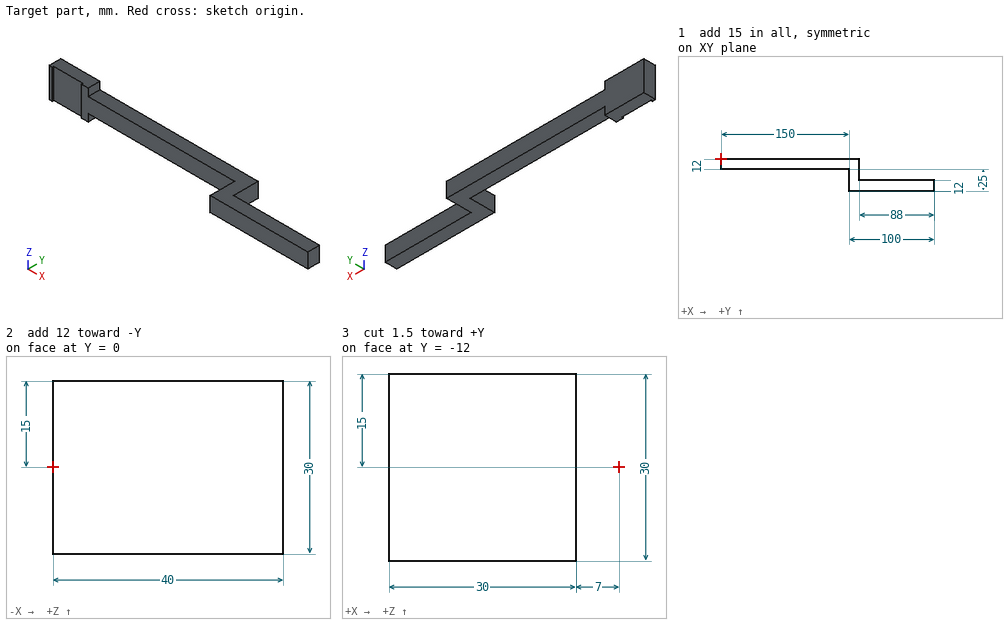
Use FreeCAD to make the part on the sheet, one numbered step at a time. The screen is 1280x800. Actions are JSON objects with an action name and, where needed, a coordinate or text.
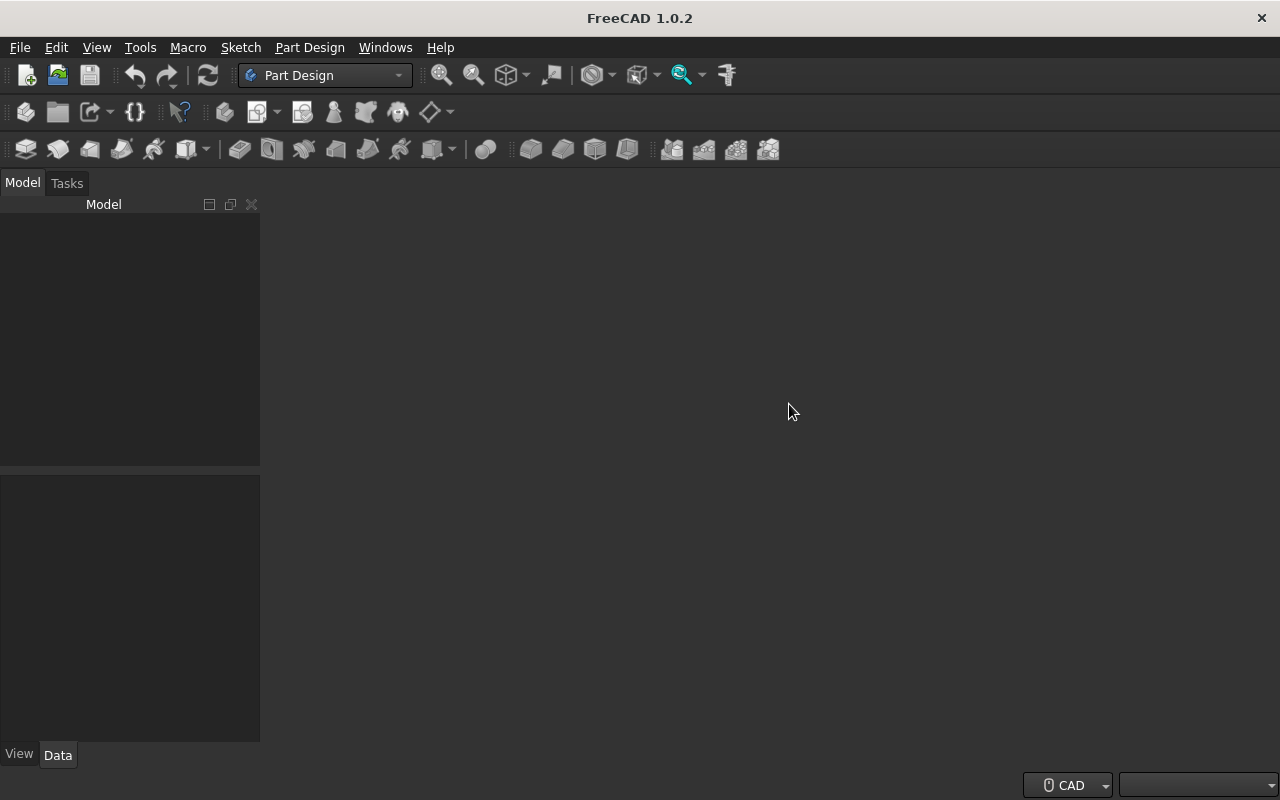
{"action": "left_click", "coordinate": [26, 76]}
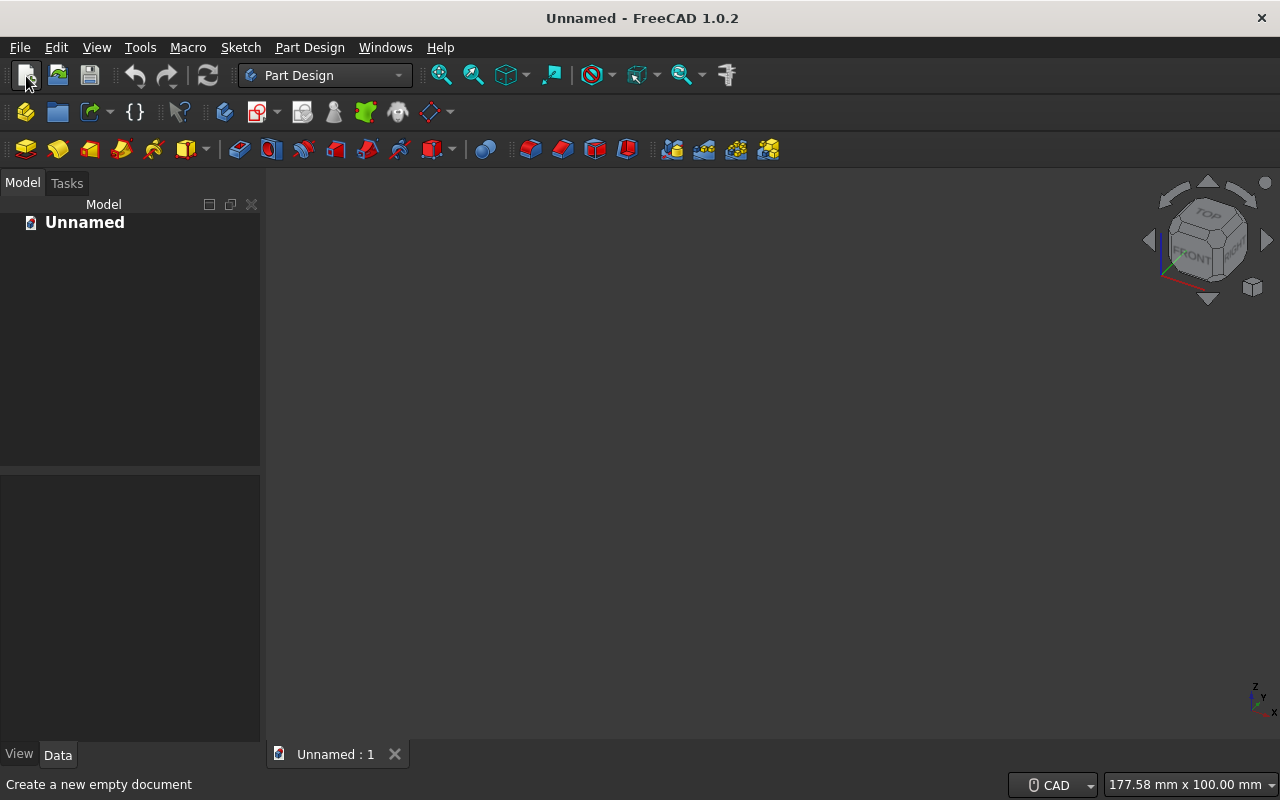
{"action": "left_click", "coordinate": [258, 112]}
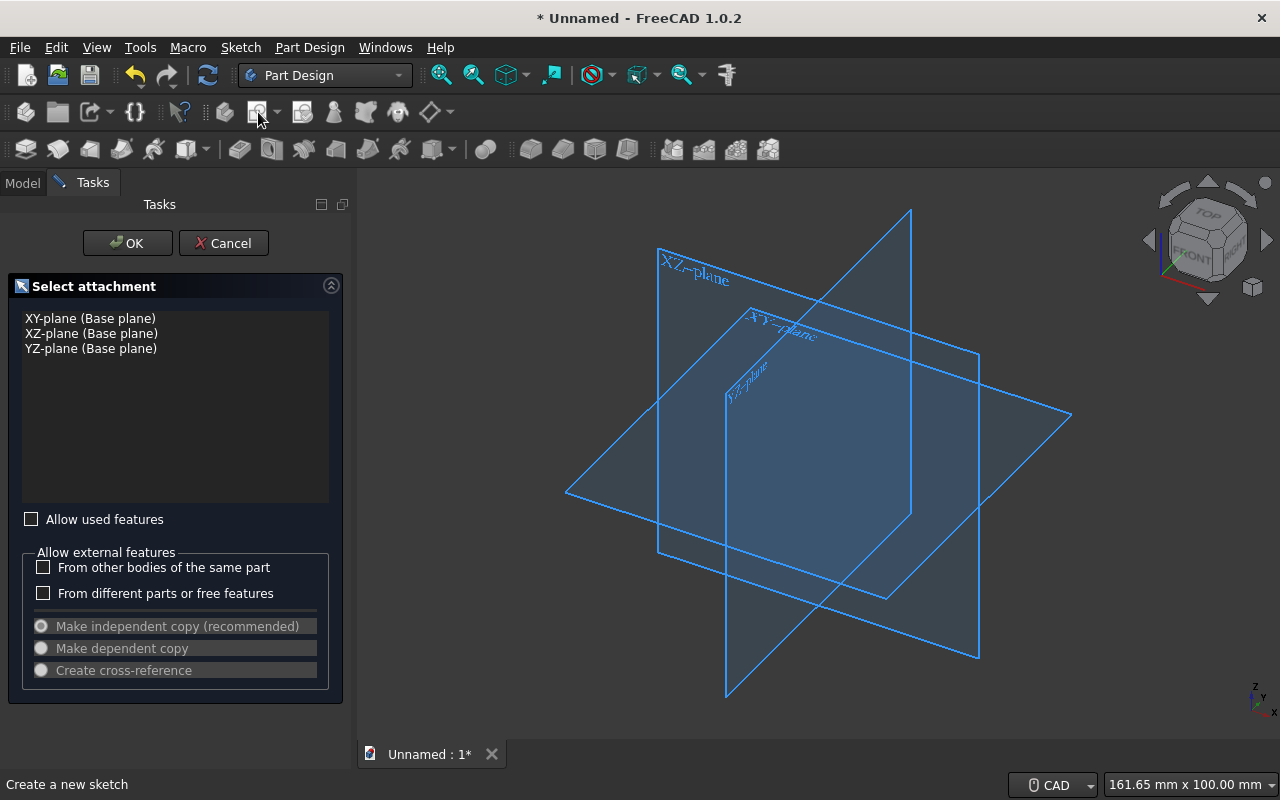
{"action": "left_click", "coordinate": [82, 318]}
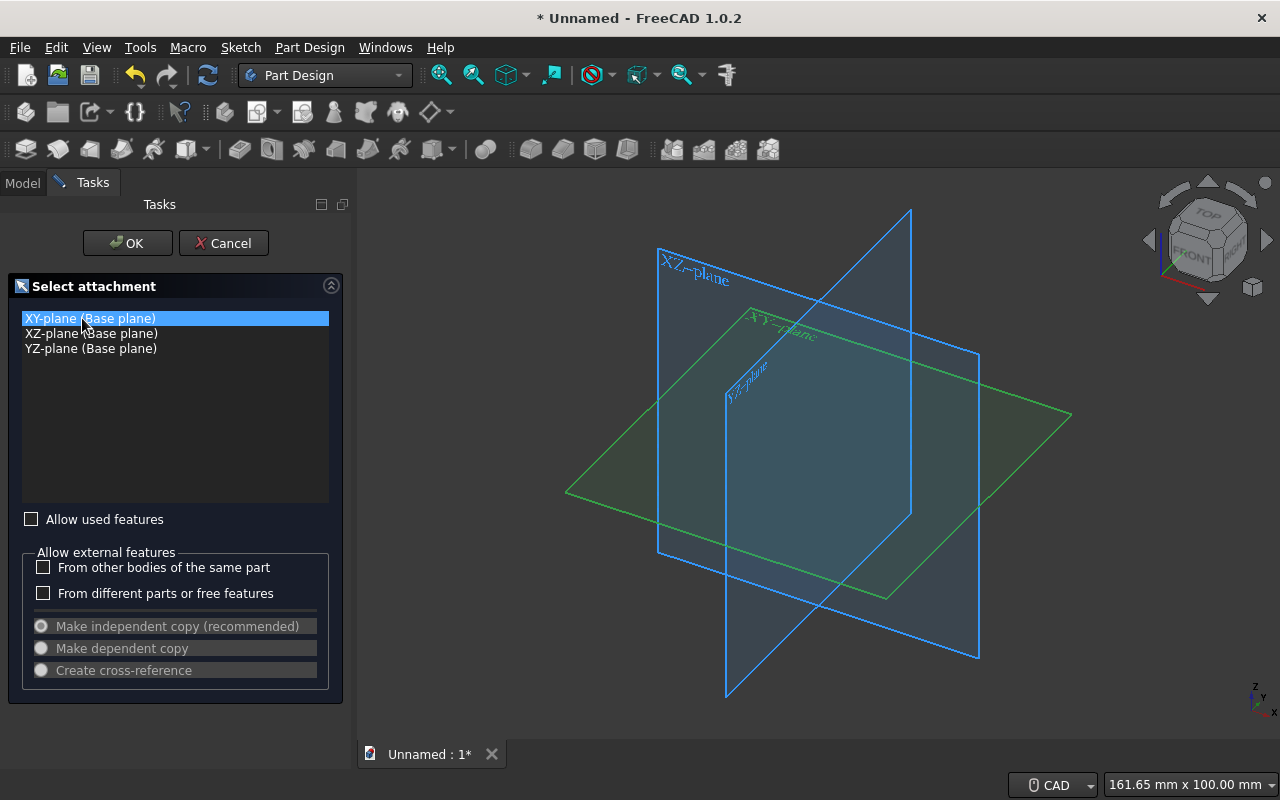
{"action": "left_click", "coordinate": [128, 243]}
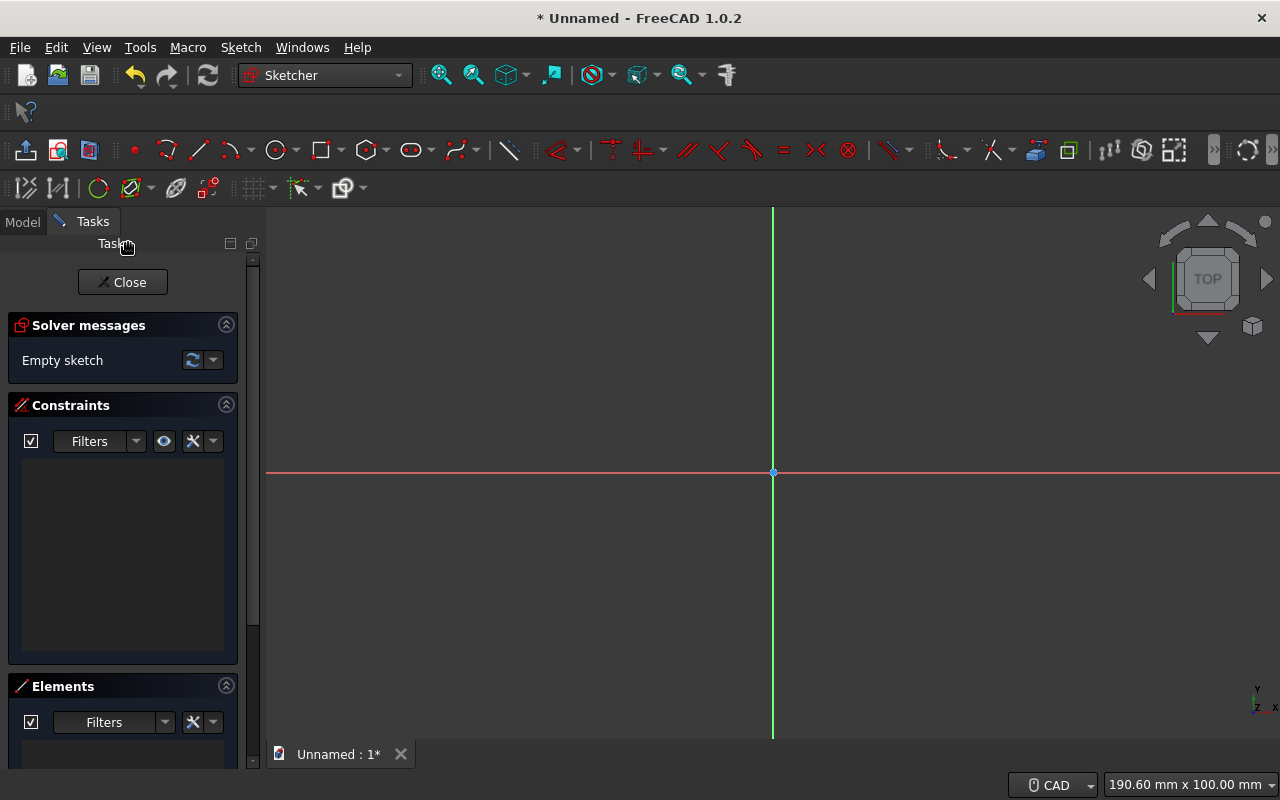
{"action": "scroll", "coordinate": [294, 416], "scroll_direction": "down", "scroll_amount": 5}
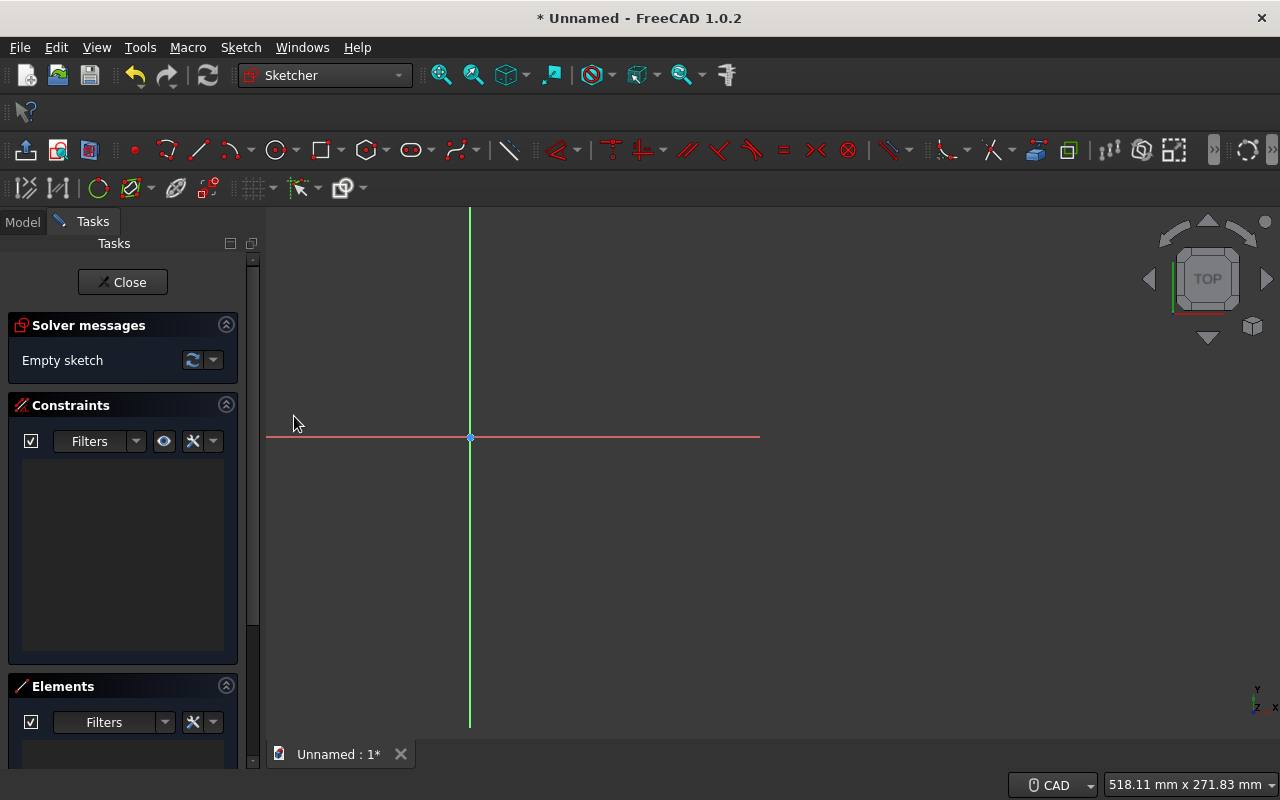
{"action": "left_click", "coordinate": [168, 150]}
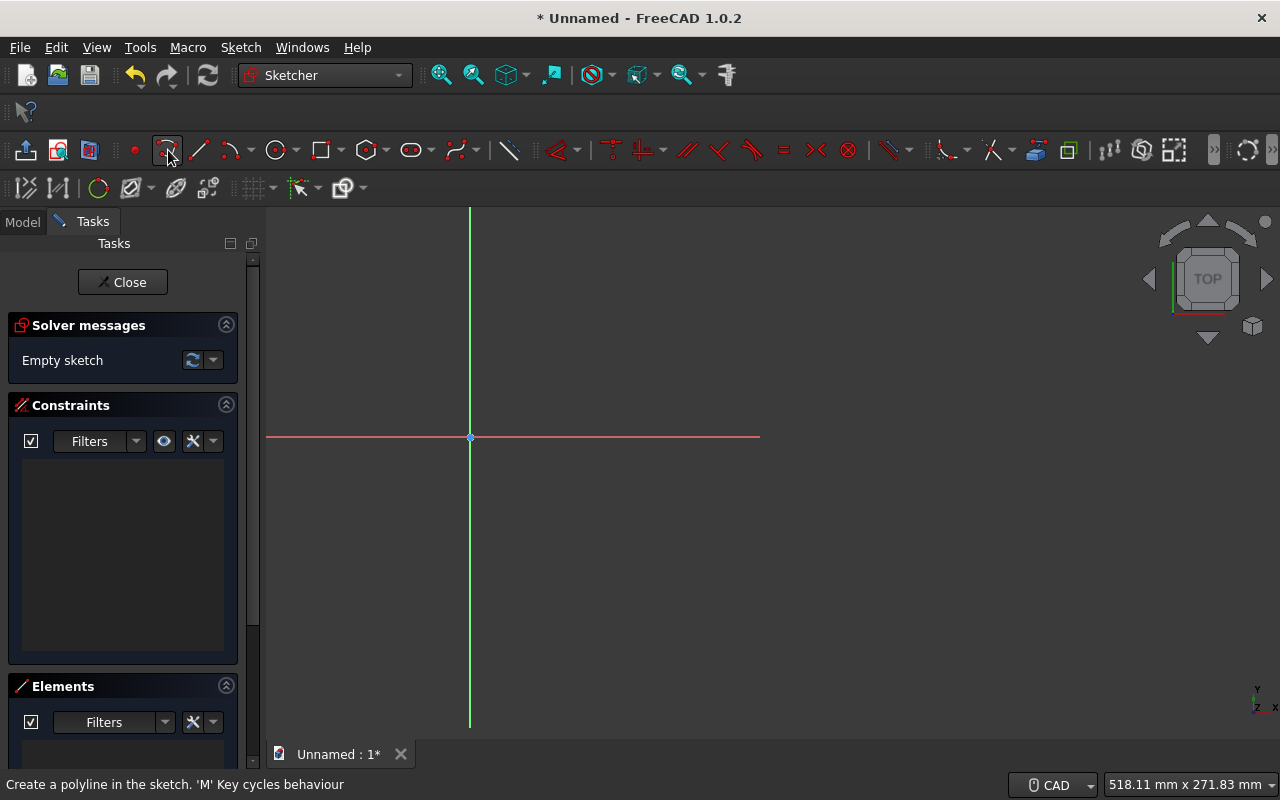
{"action": "left_click", "coordinate": [470, 437]}
{"action": "left_click", "coordinate": [479, 461]}
{"action": "left_click", "coordinate": [764, 461]}
{"action": "left_click", "coordinate": [764, 510]}
{"action": "left_click", "coordinate": [960, 510]}
{"action": "left_click", "coordinate": [960, 486]}
{"action": "left_click", "coordinate": [787, 486]}
{"action": "left_click", "coordinate": [787, 446]}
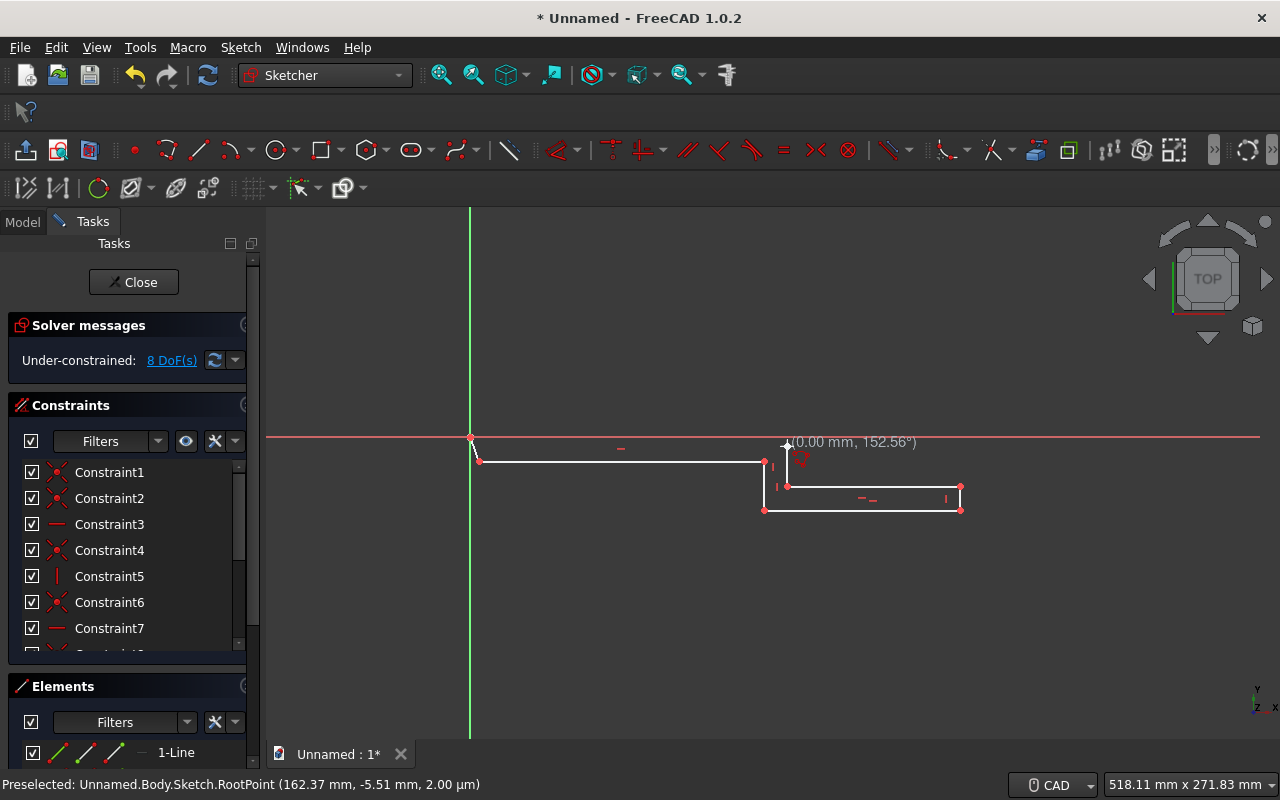
{"action": "scroll", "coordinate": [470, 437], "scroll_direction": "up", "scroll_amount": 2}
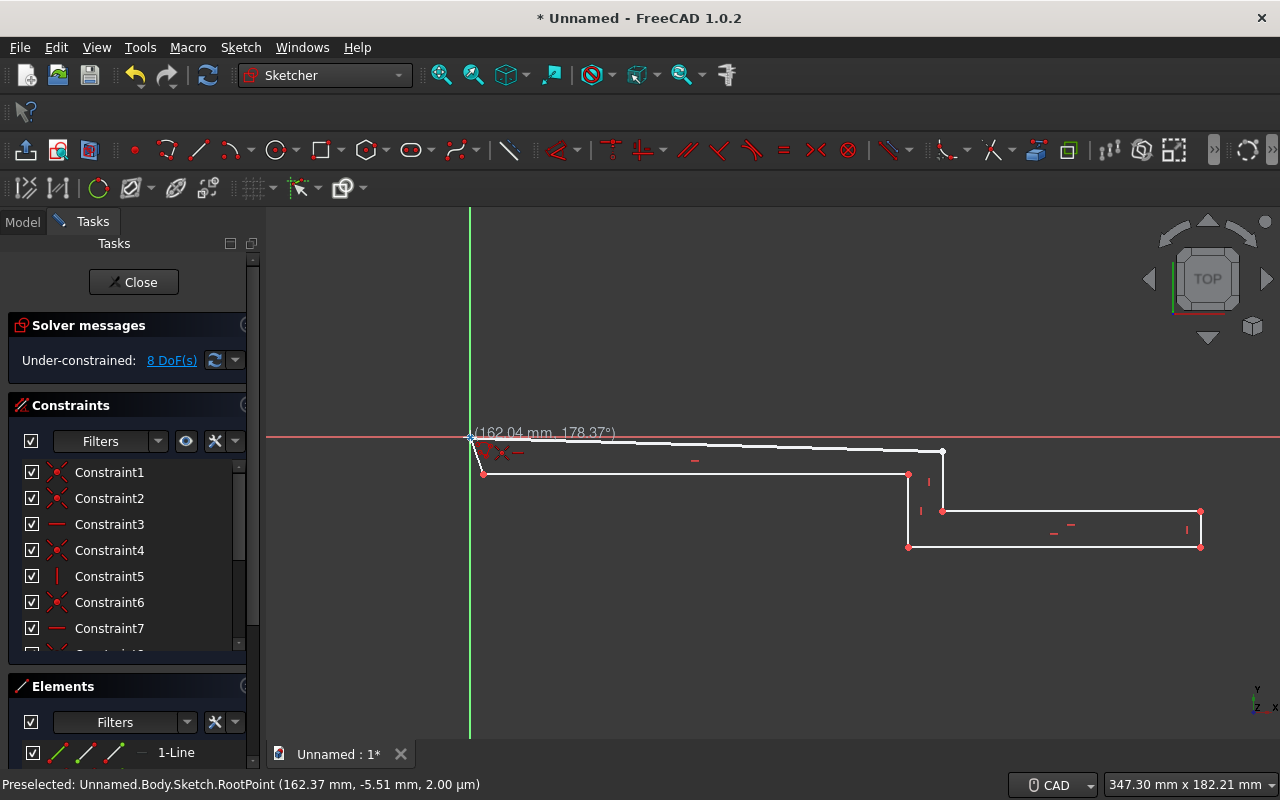
{"action": "left_click", "coordinate": [470, 437]}
{"action": "key", "text": "Escape"}
{"action": "key", "text": "Escape"}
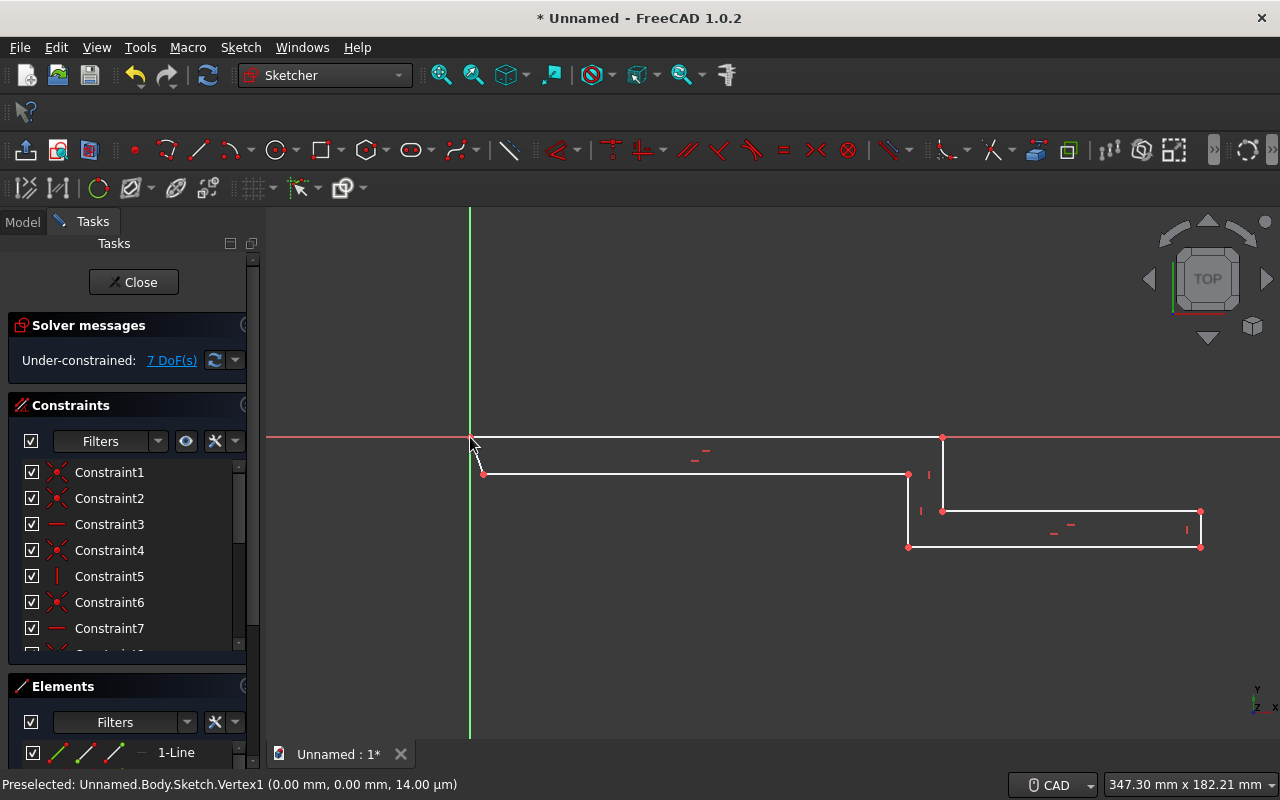
{"action": "scroll", "coordinate": [474, 448], "scroll_direction": "up", "scroll_amount": 2}